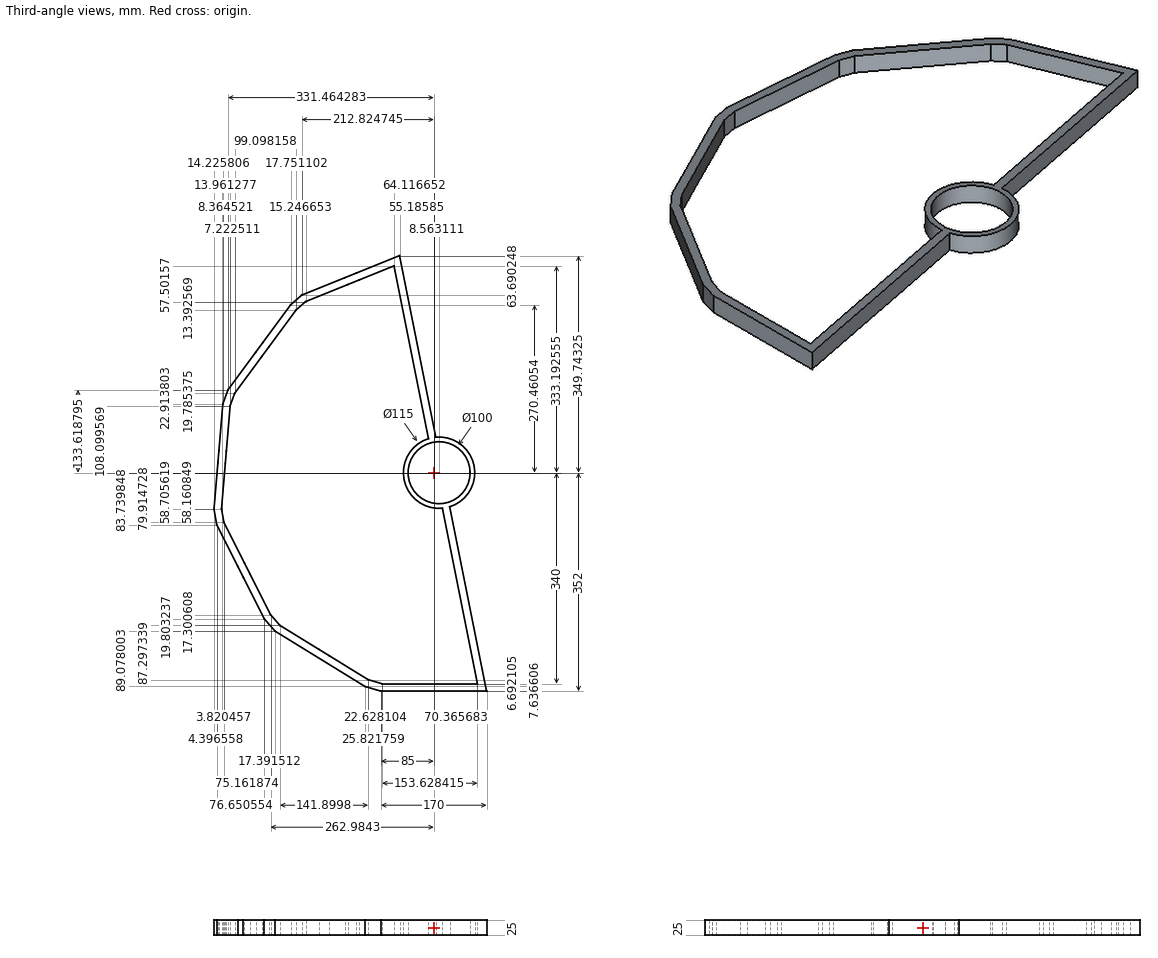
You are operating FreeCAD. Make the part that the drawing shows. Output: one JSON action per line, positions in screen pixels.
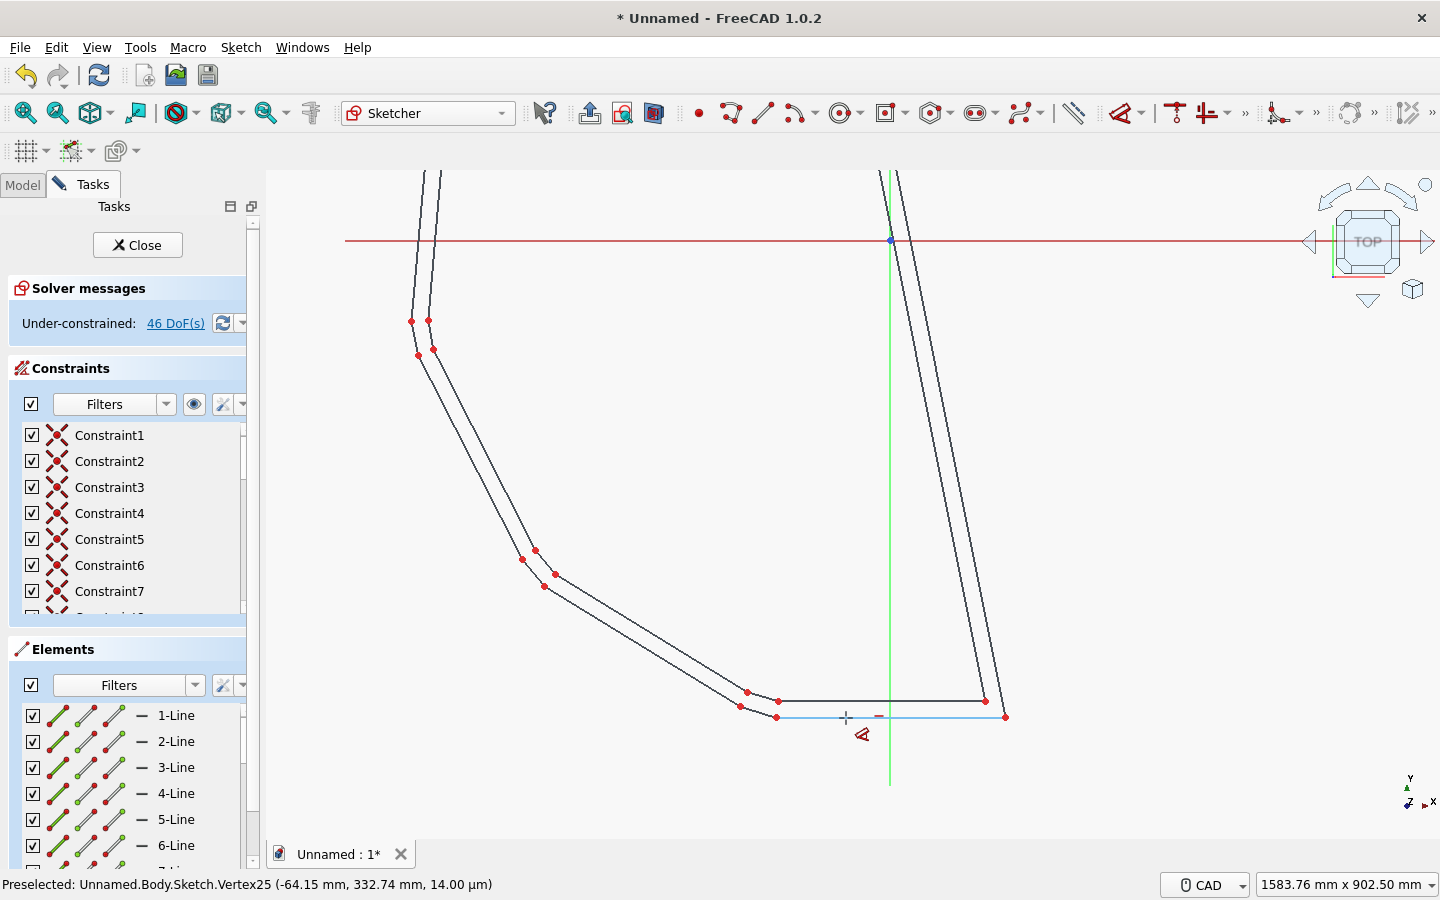
{"action": "left_click", "coordinate": [845, 718]}
{"action": "left_click", "coordinate": [838, 752]}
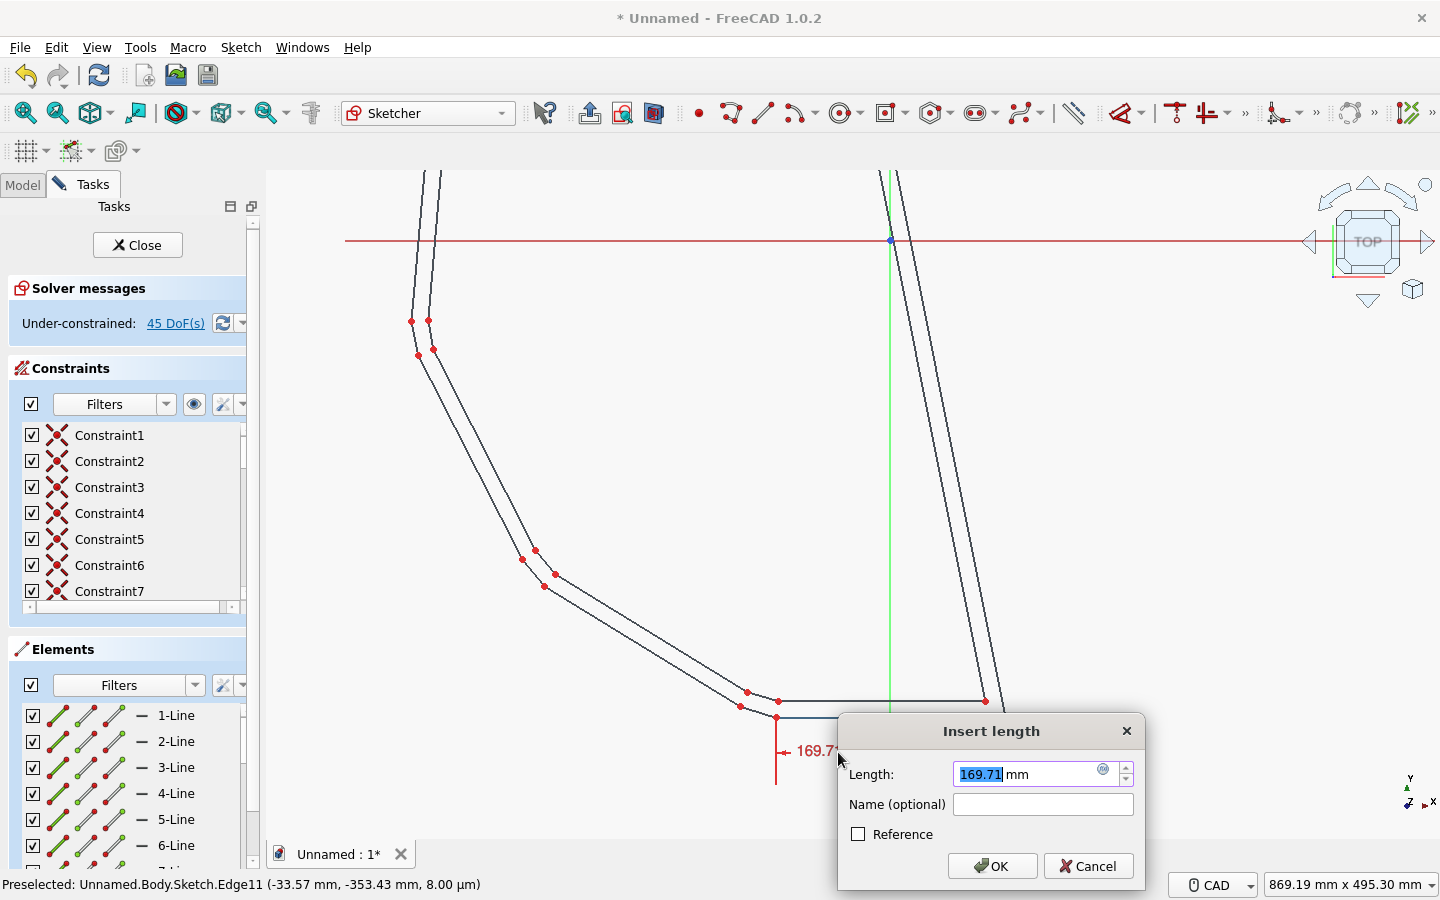
{"action": "type", "text": "170"}
{"action": "key", "text": "Return"}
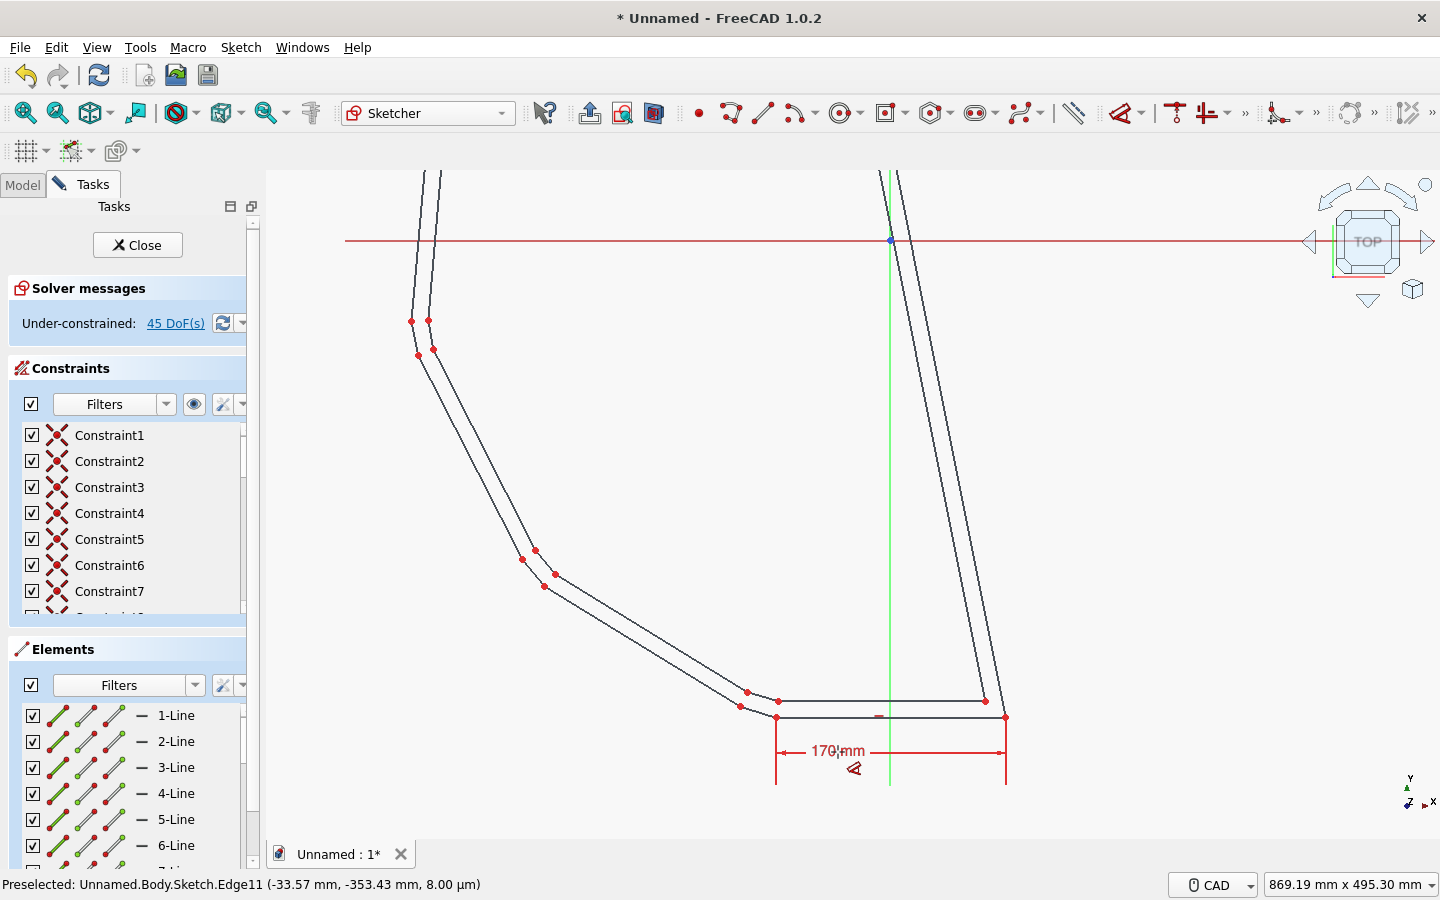
{"action": "left_click", "coordinate": [776, 718]}
{"action": "left_click", "coordinate": [833, 207]}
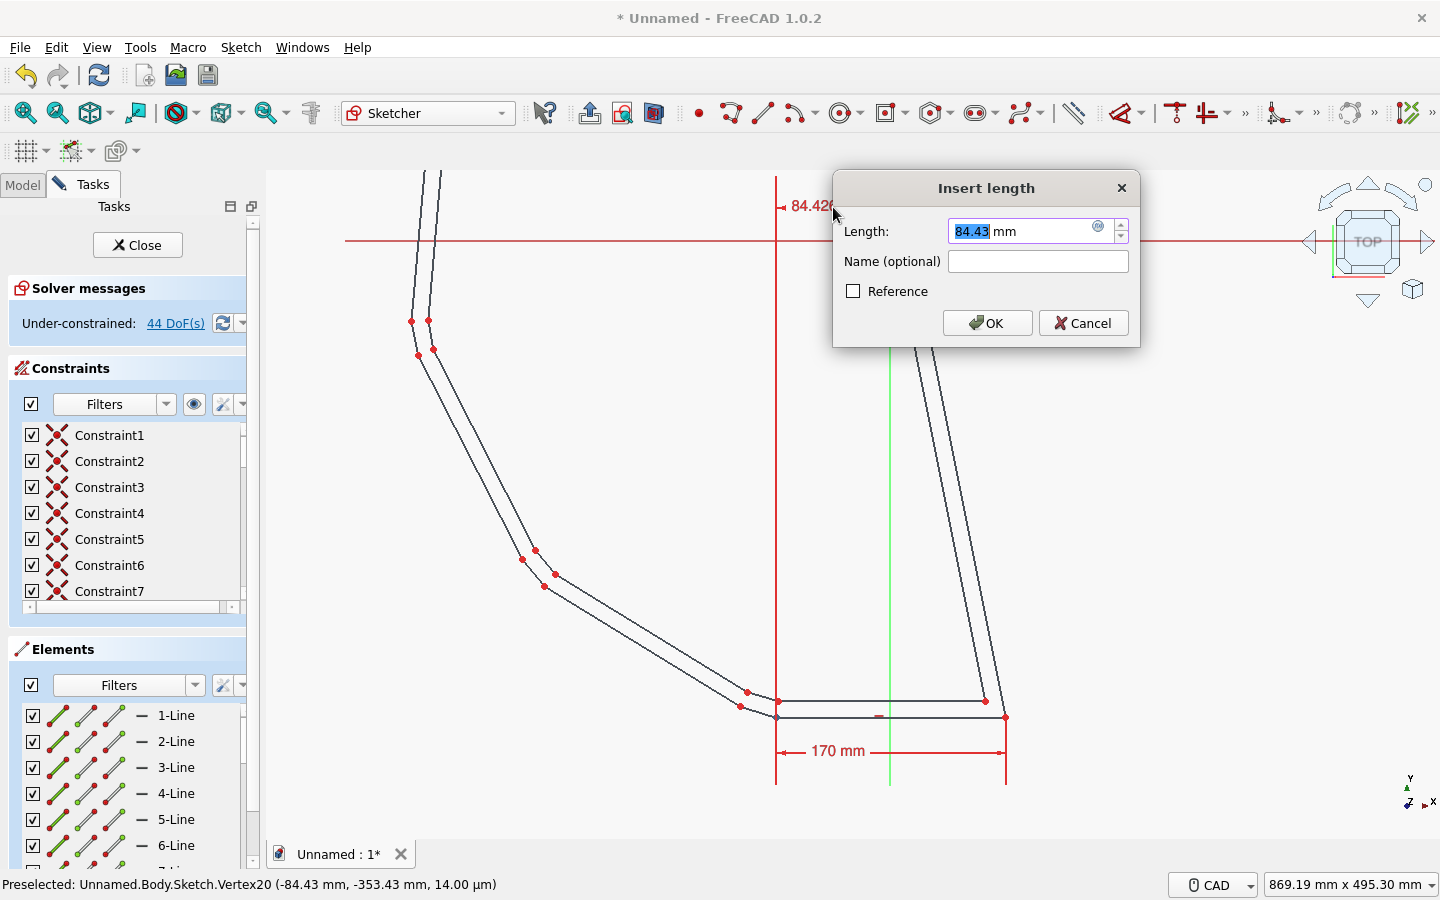
{"action": "type", "text": "85"}
{"action": "key", "text": "Return"}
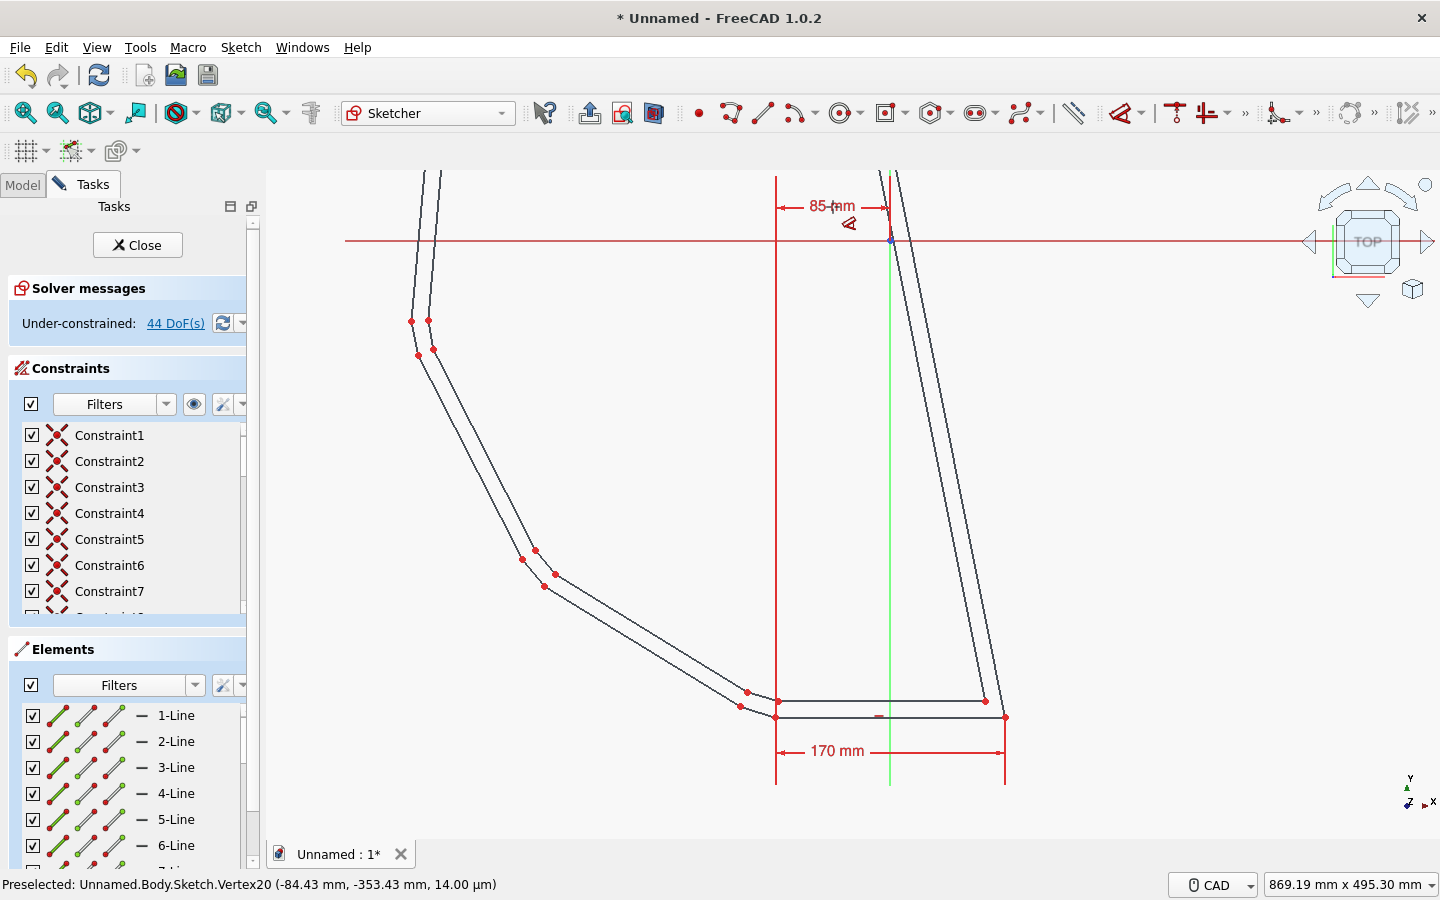
{"action": "left_click", "coordinate": [776, 718]}
{"action": "left_click", "coordinate": [924, 479]}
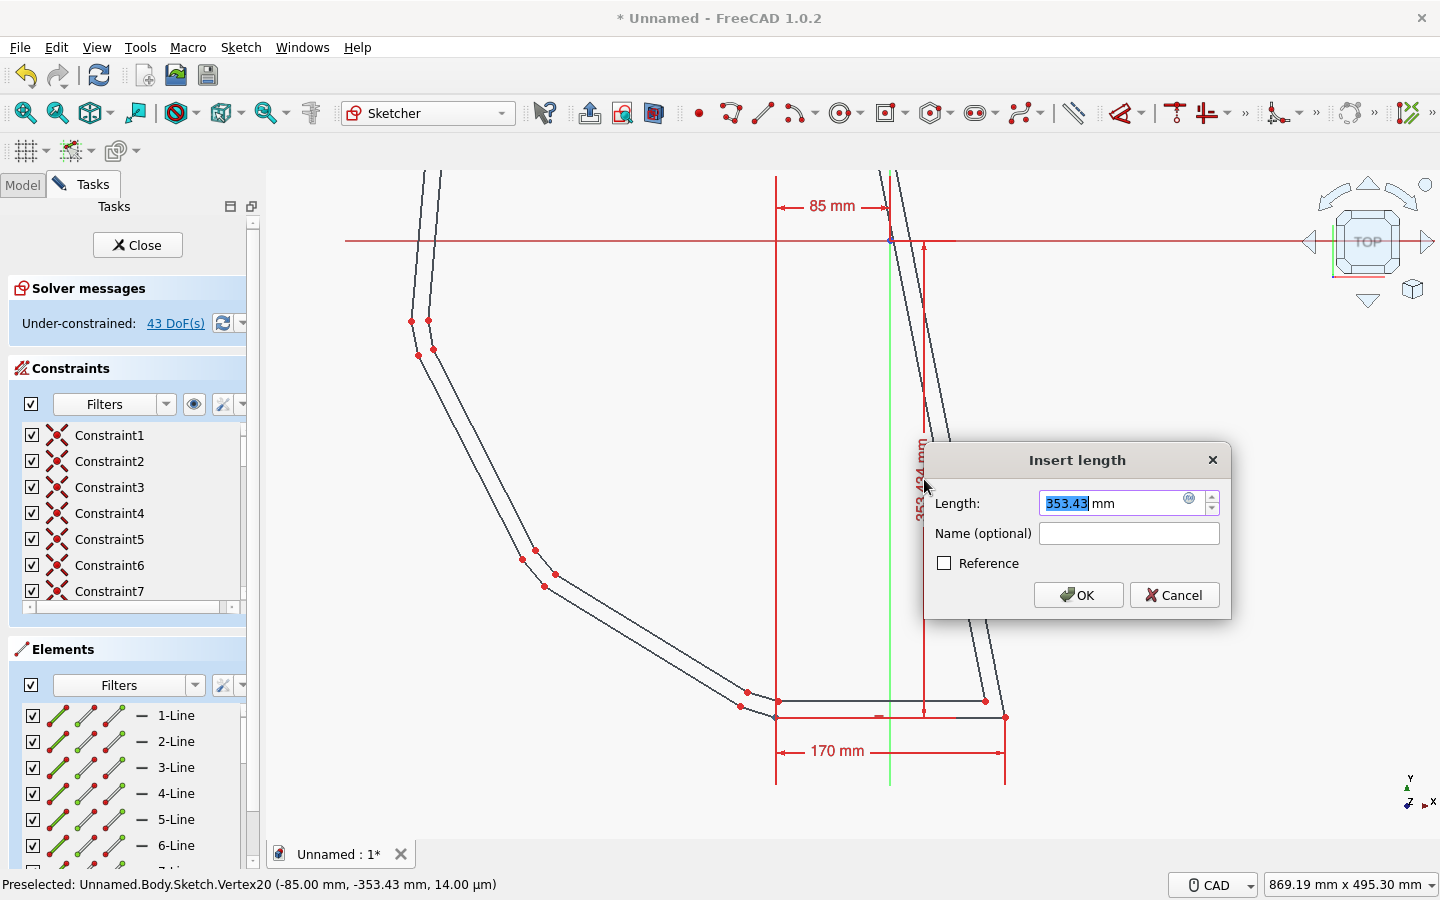
{"action": "type", "text": "352"}
{"action": "key", "text": "Return"}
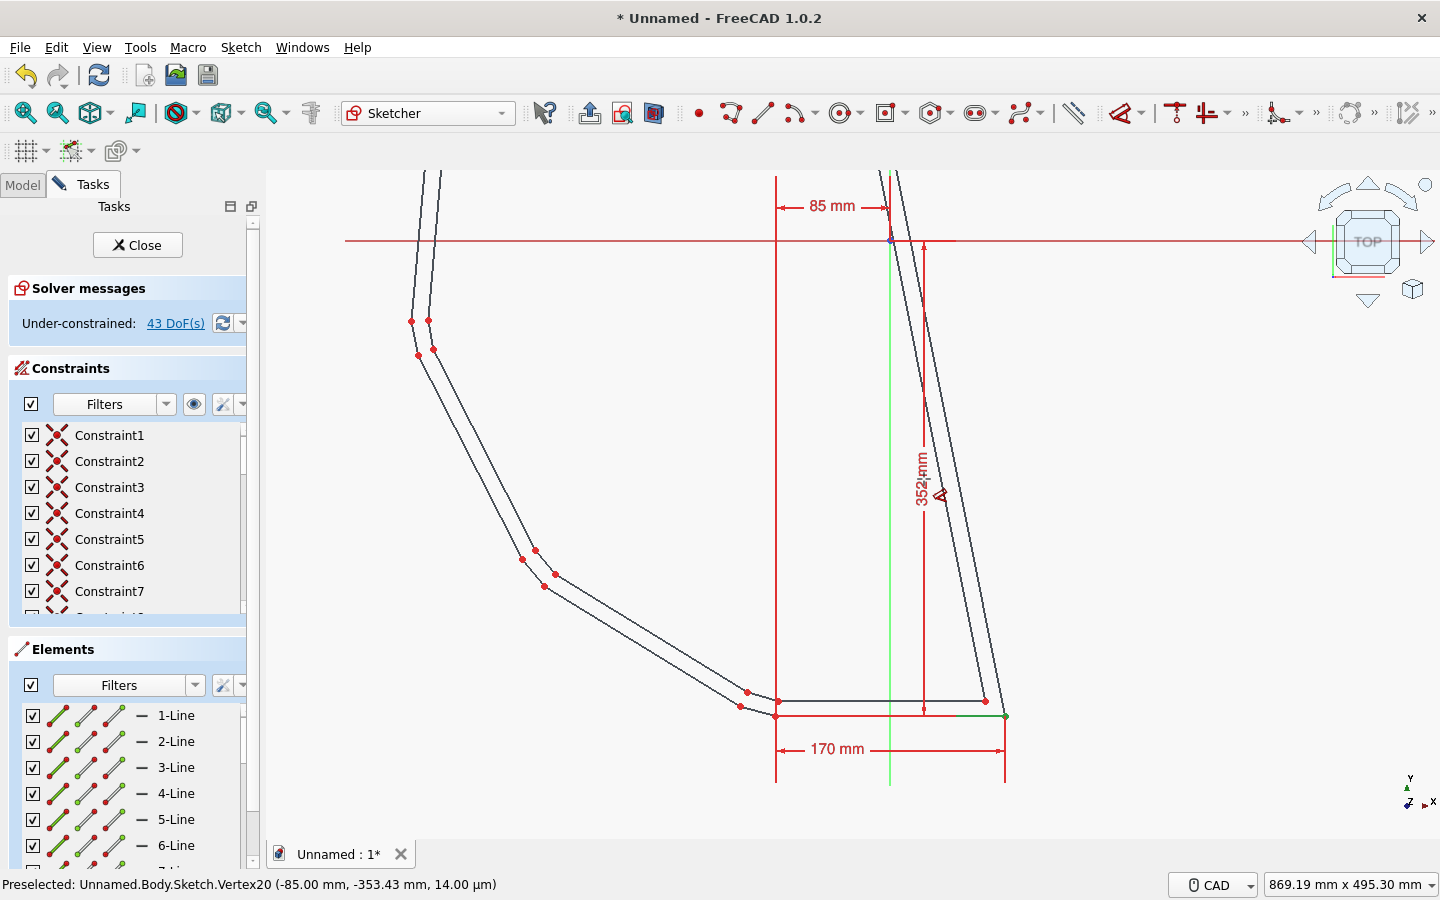
{"action": "left_click", "coordinate": [985, 701]}
{"action": "left_click", "coordinate": [1019, 471]}